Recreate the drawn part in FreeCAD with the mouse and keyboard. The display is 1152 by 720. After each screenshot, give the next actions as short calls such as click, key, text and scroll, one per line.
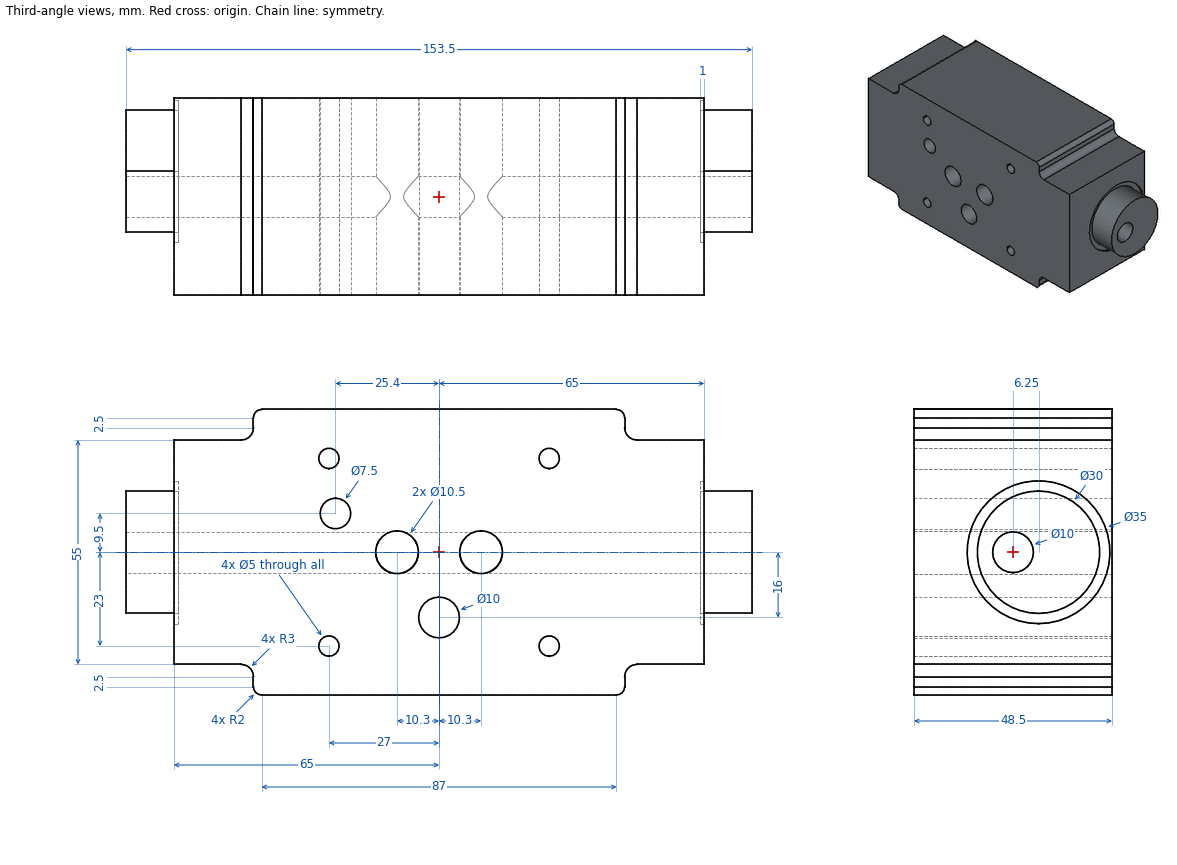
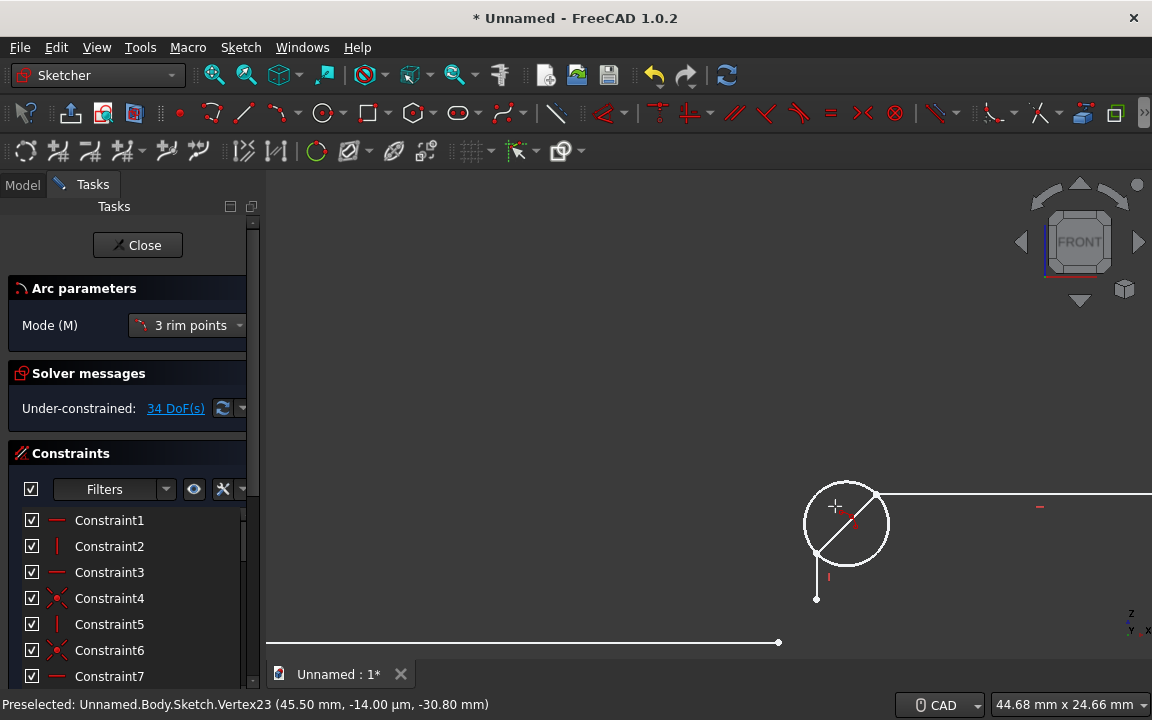
click(834, 506)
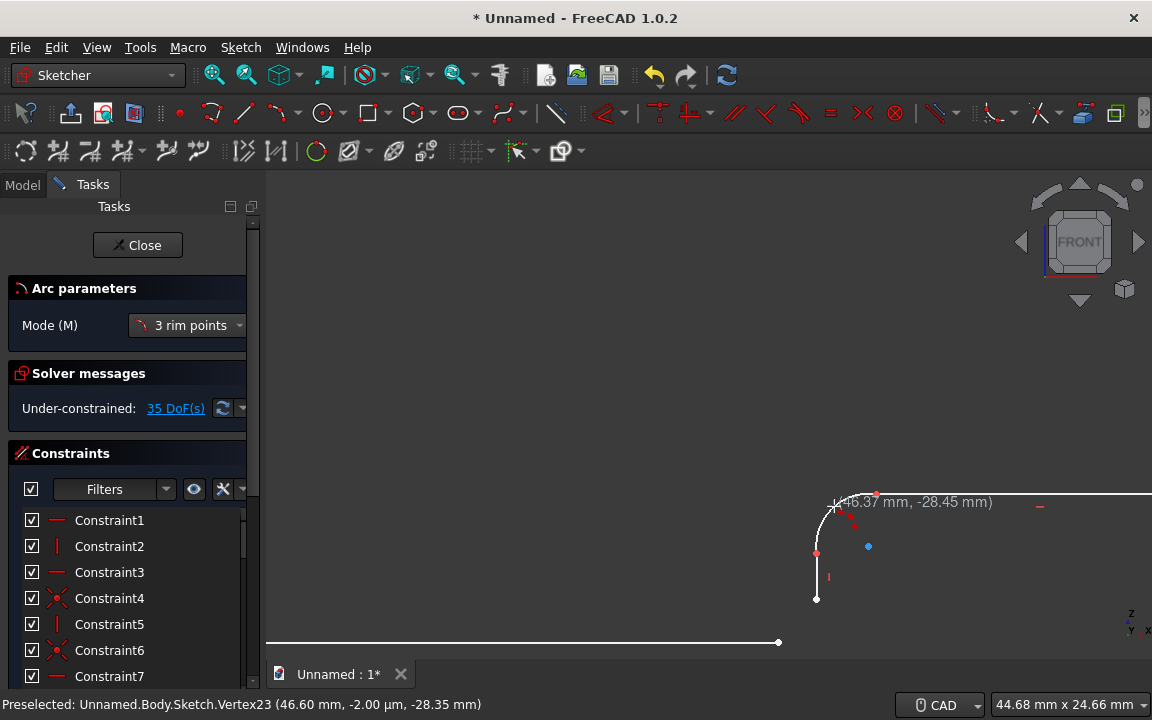
click(817, 600)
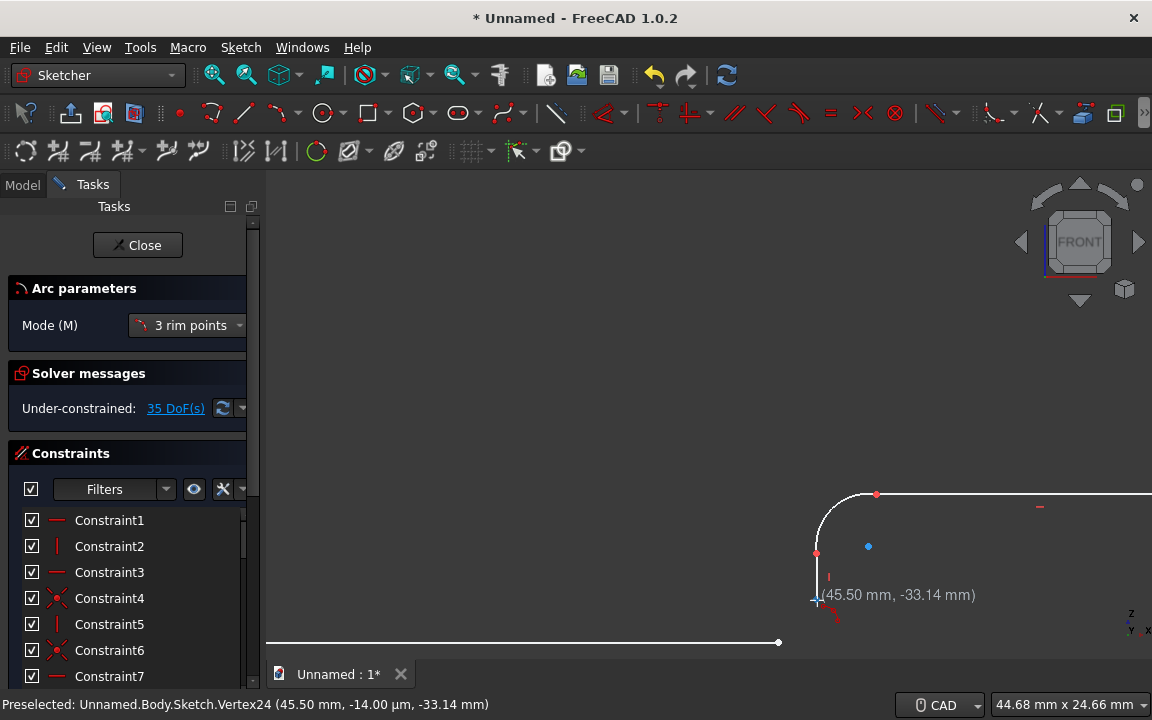
scroll(824, 534, down, 8)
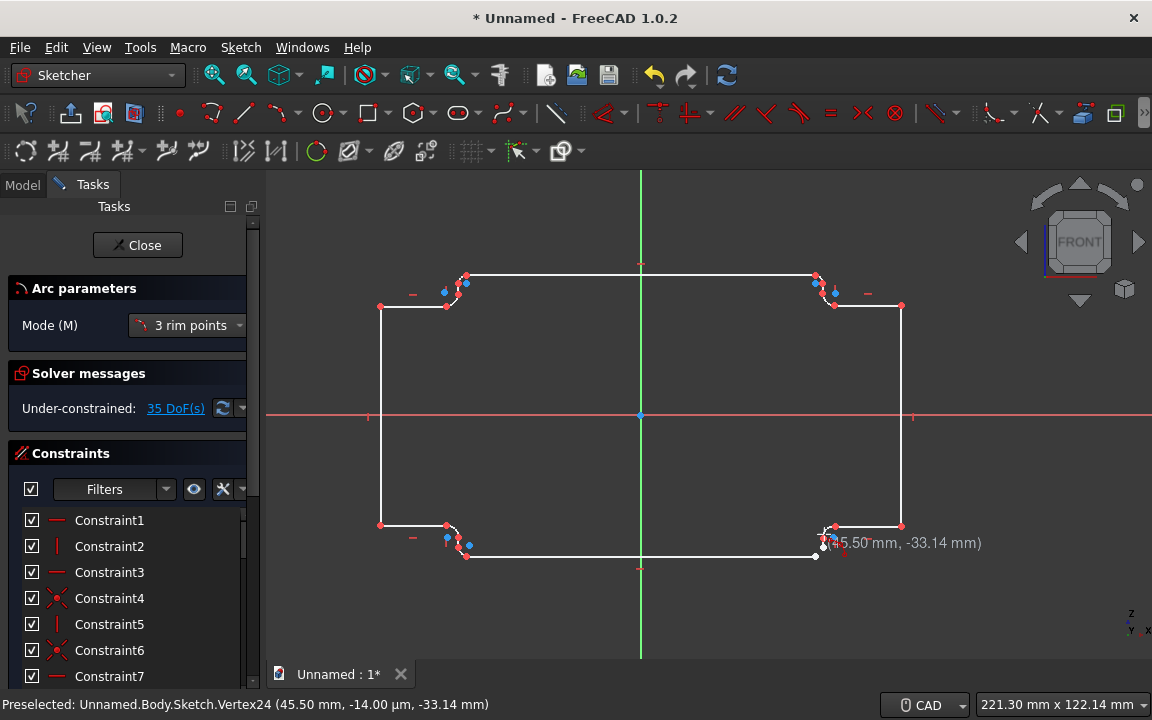
scroll(815, 555, up, 2)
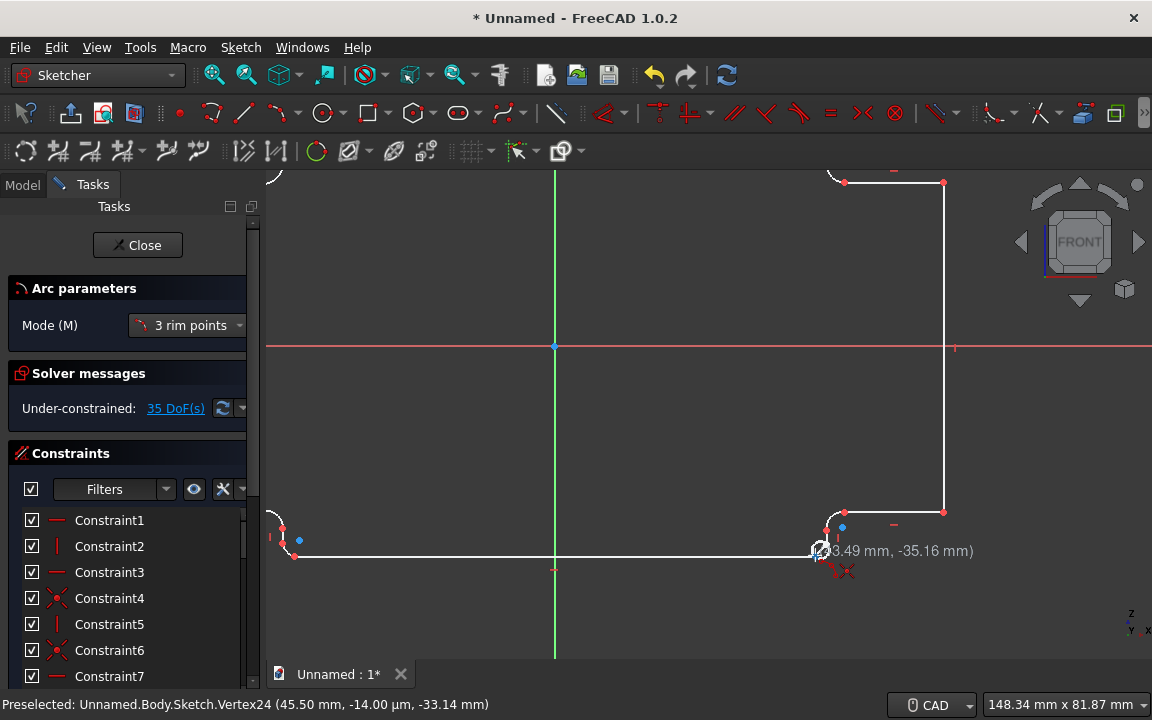
click(815, 557)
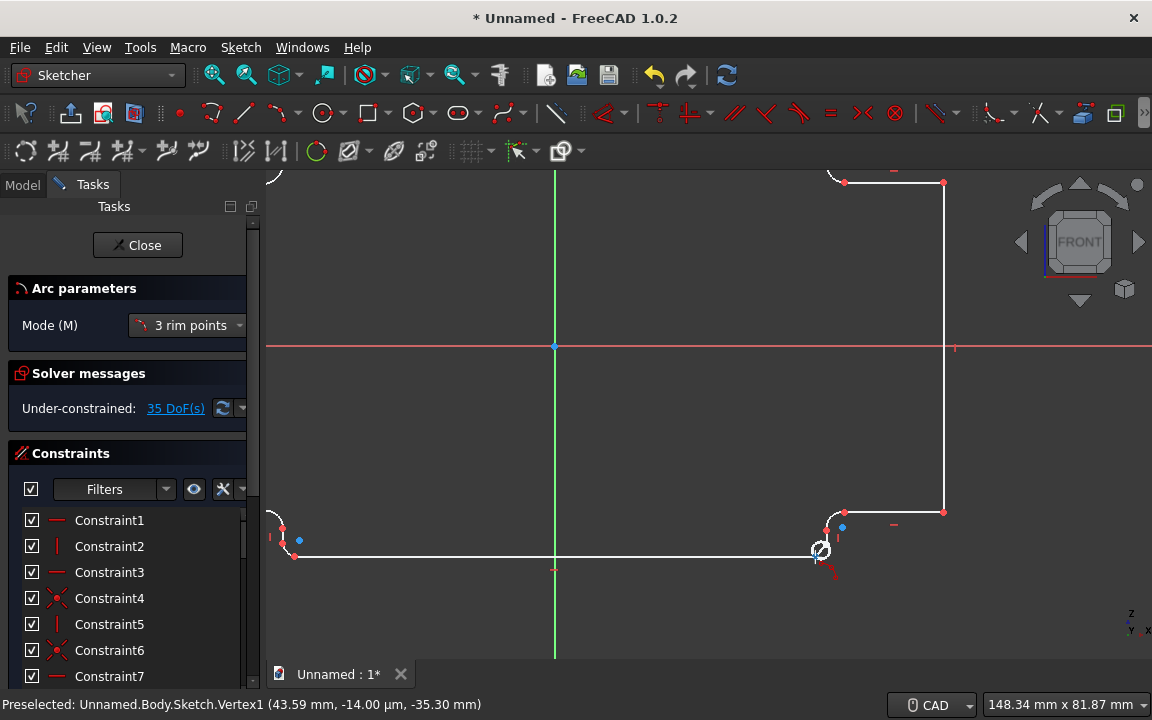
scroll(823, 552, up, 8)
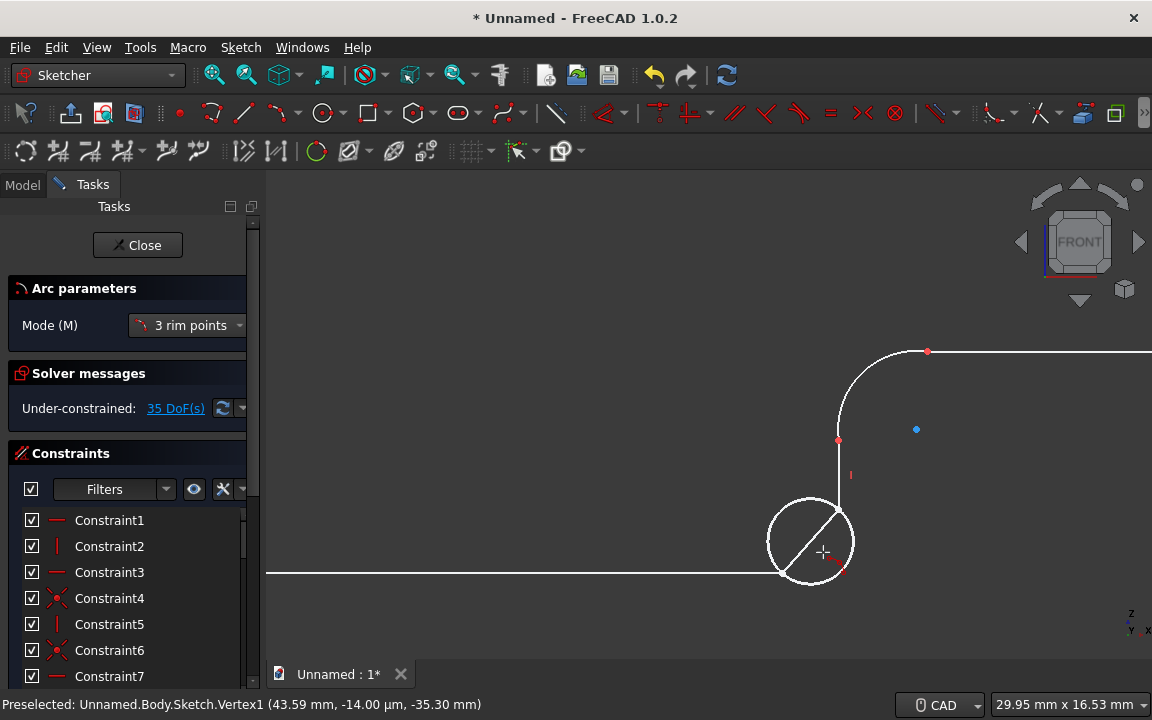
click(822, 547)
key(Escape)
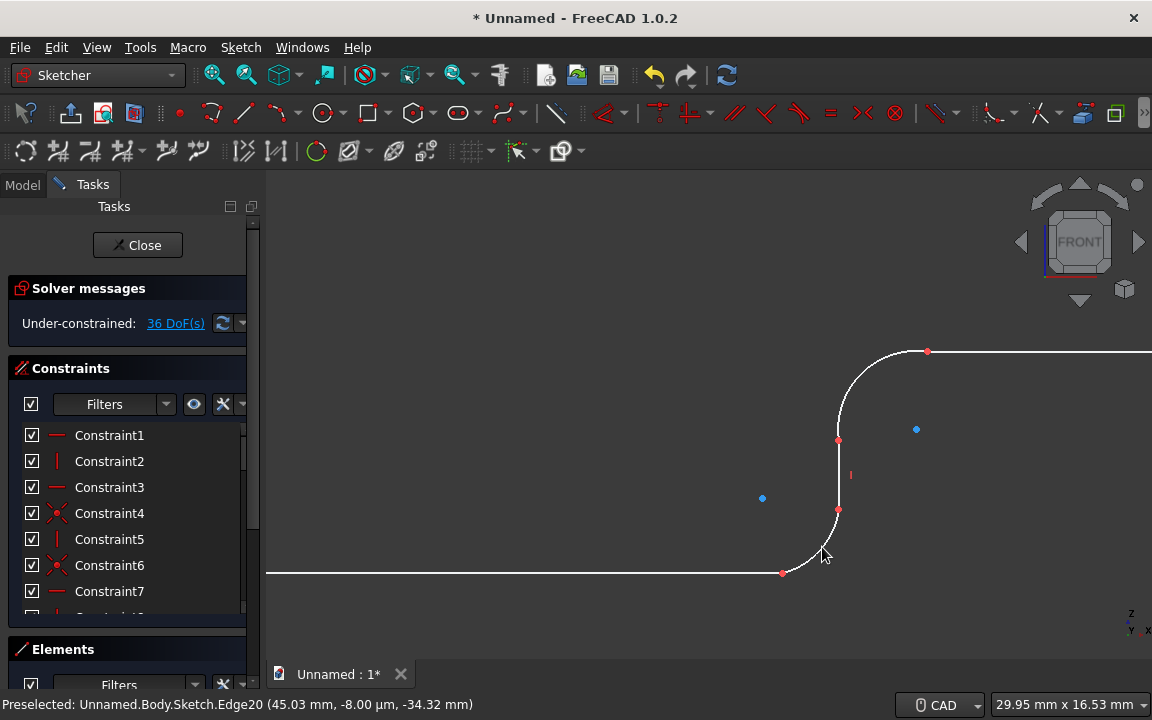
scroll(820, 553, down, 10)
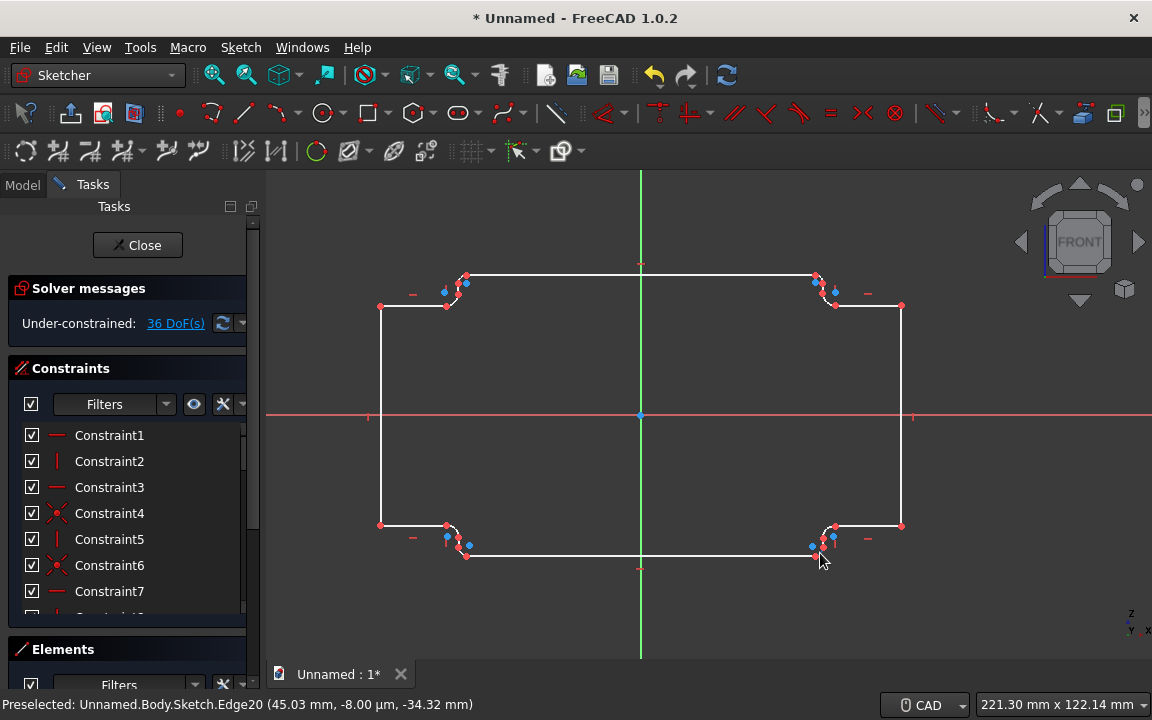
click(711, 556)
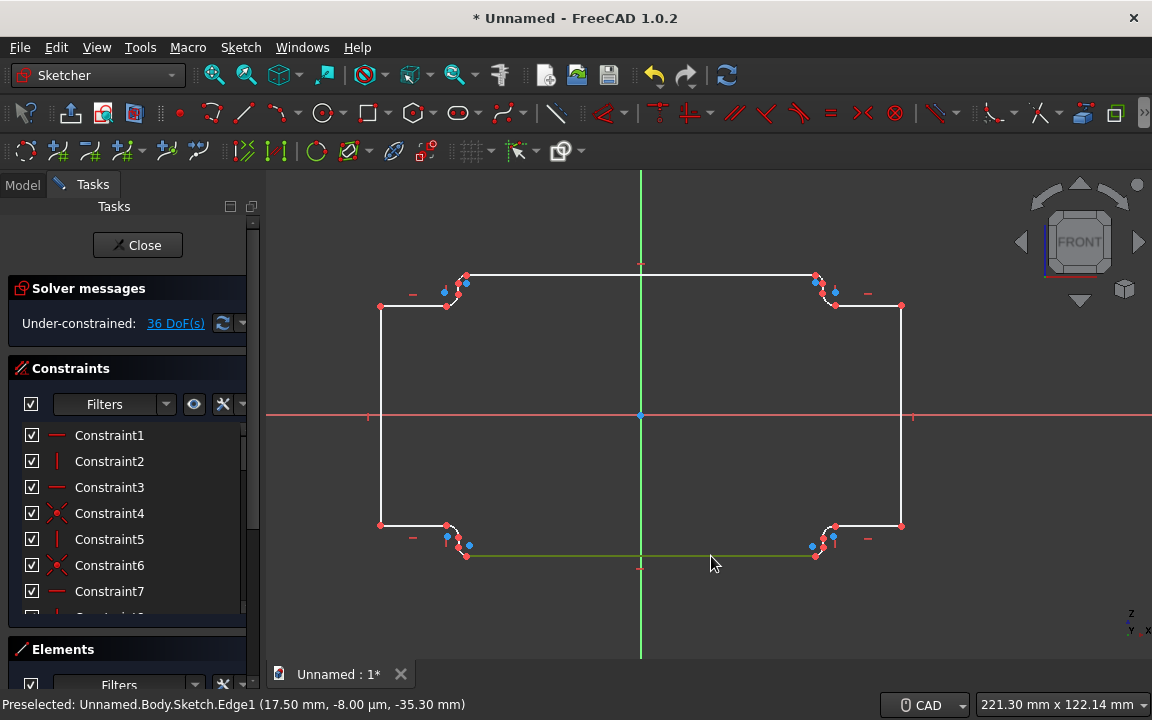
scroll(461, 553, up, 5)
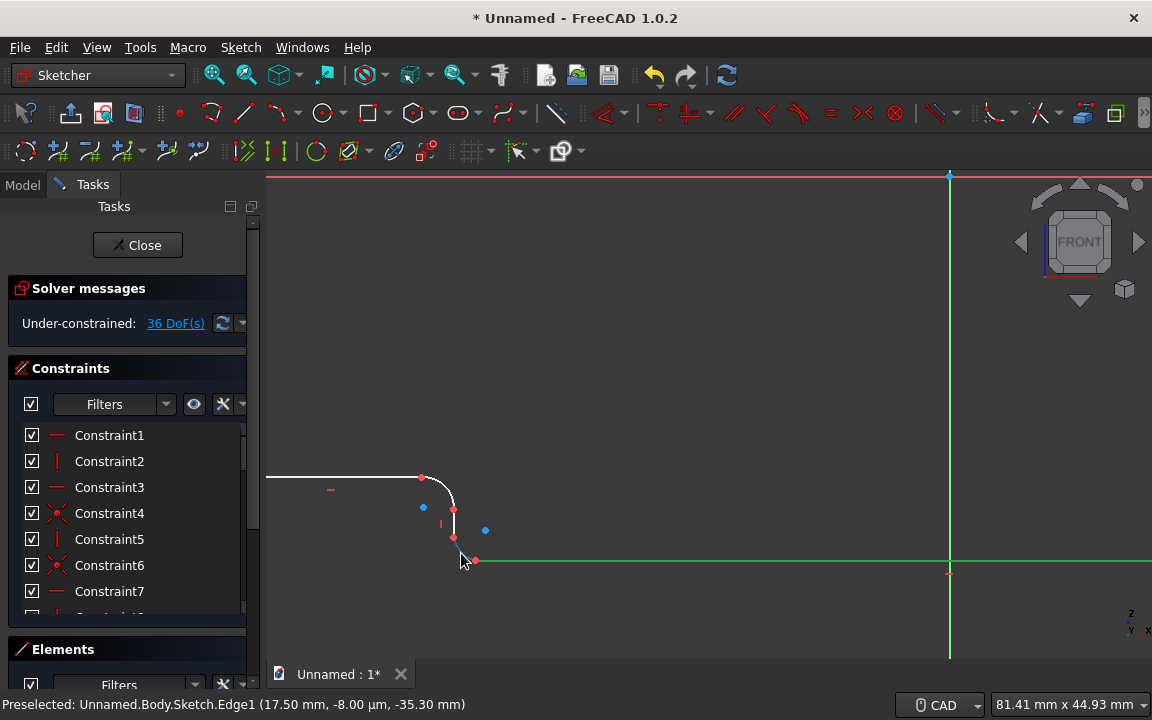
click(461, 552)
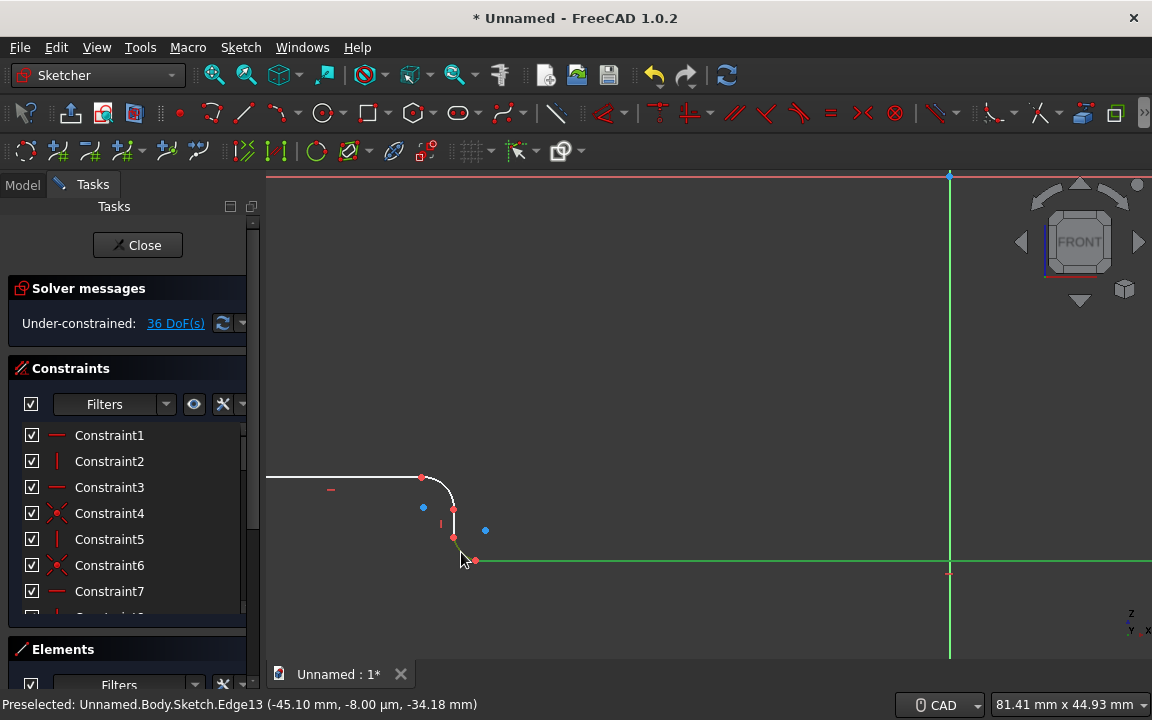
click(800, 114)